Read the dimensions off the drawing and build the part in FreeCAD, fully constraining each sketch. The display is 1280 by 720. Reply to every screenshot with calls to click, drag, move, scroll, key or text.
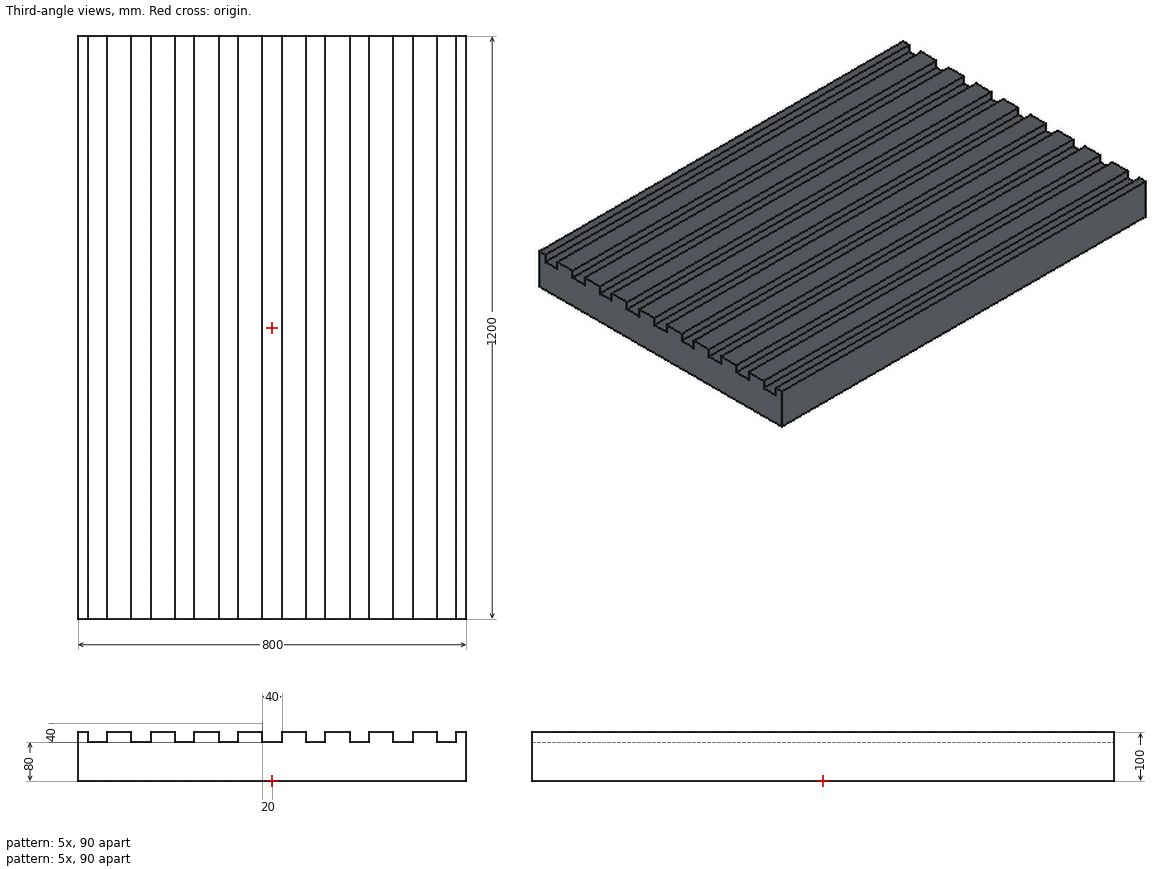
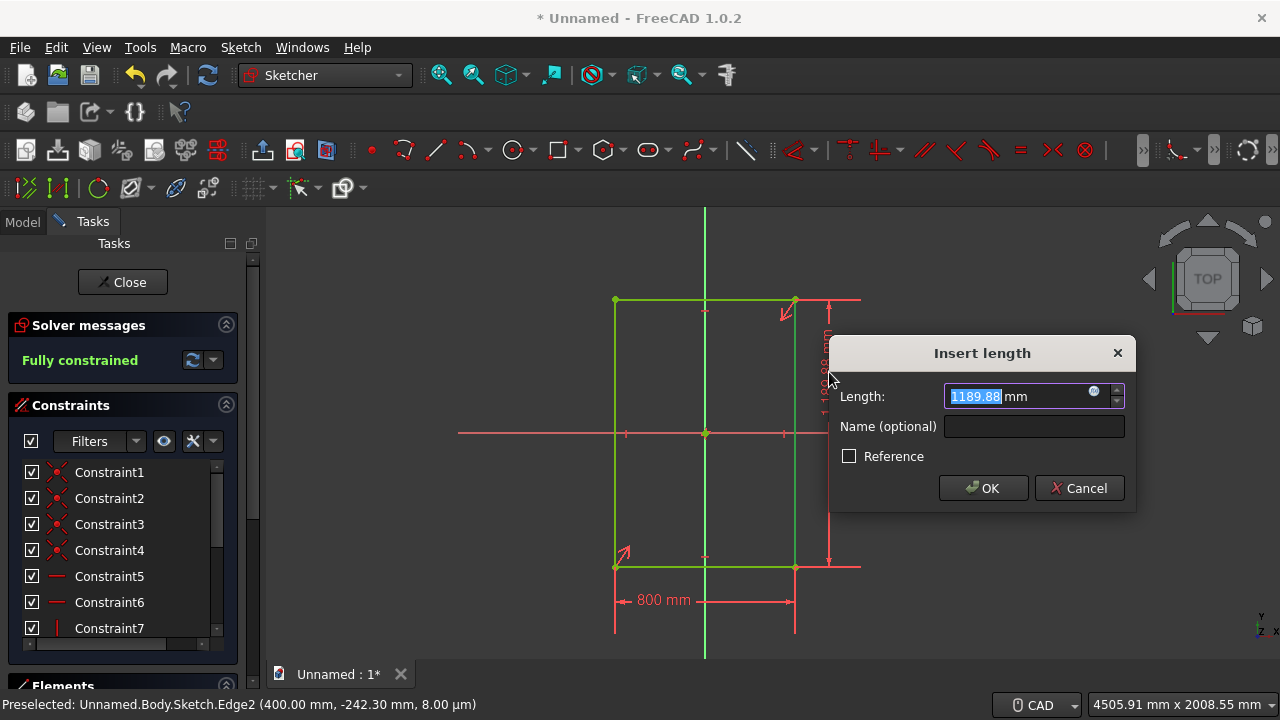
text(1200)
key(Return)
key(Escape)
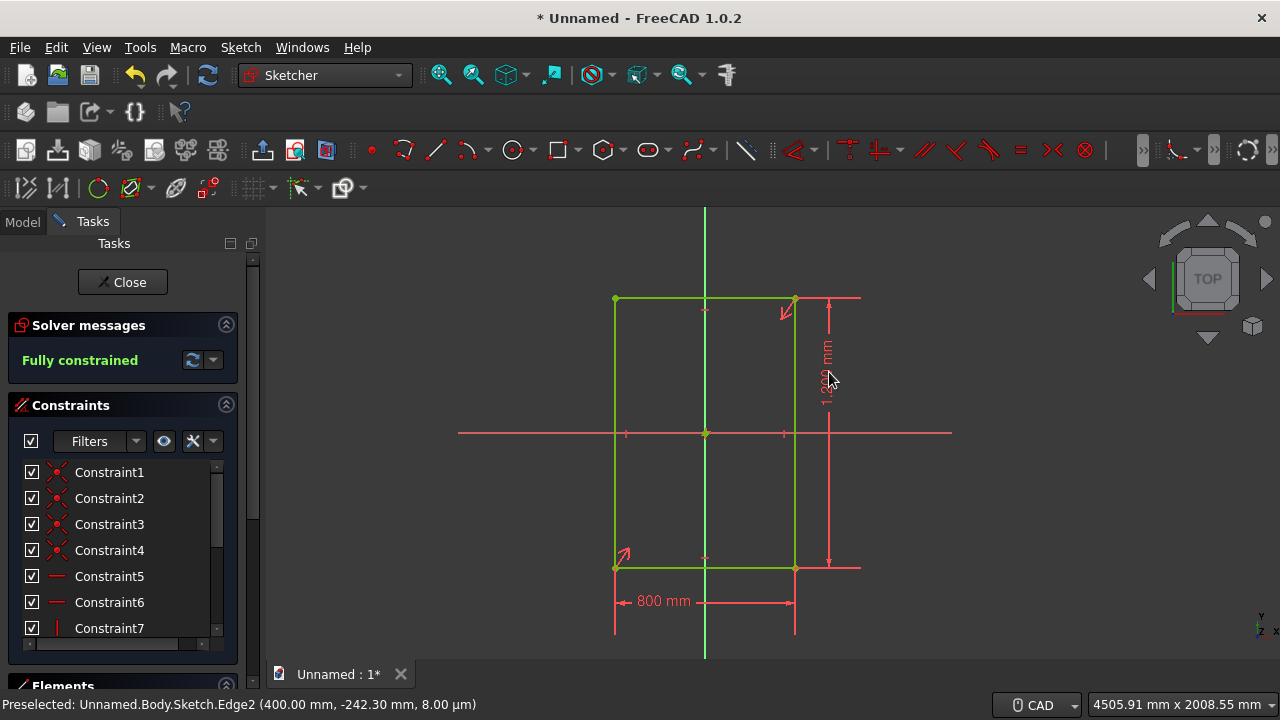
click(123, 282)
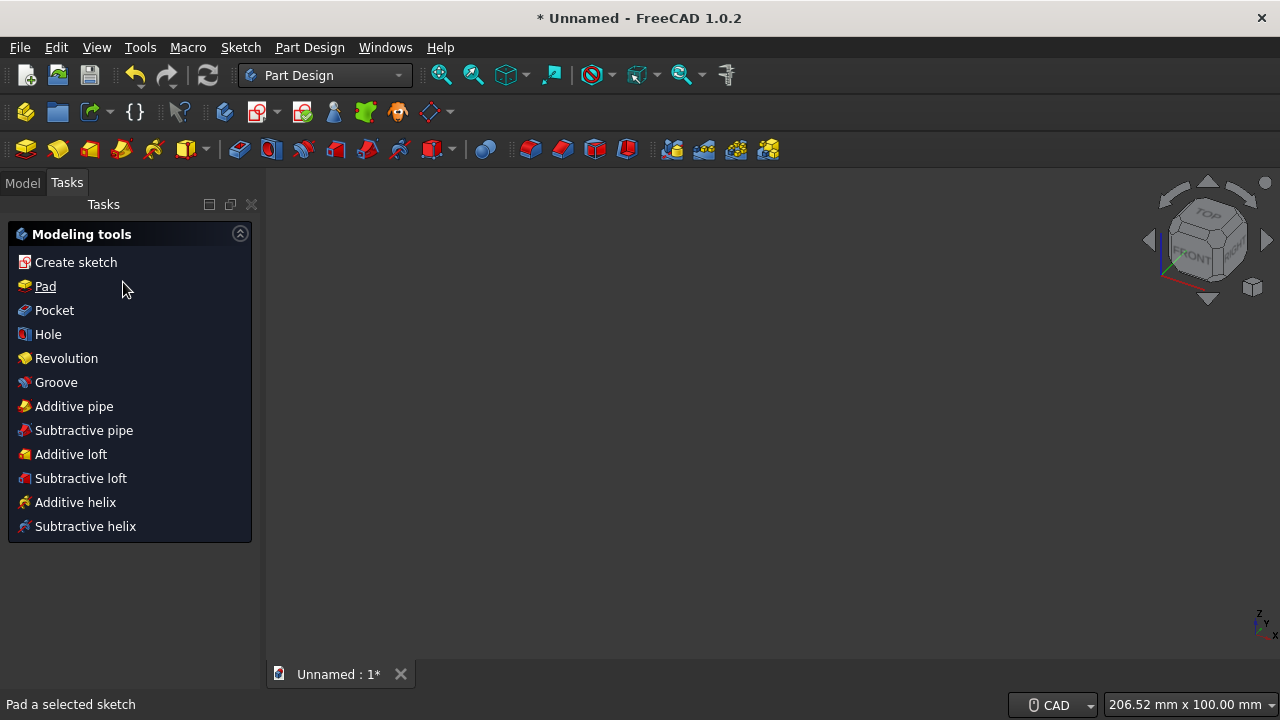
click(26, 150)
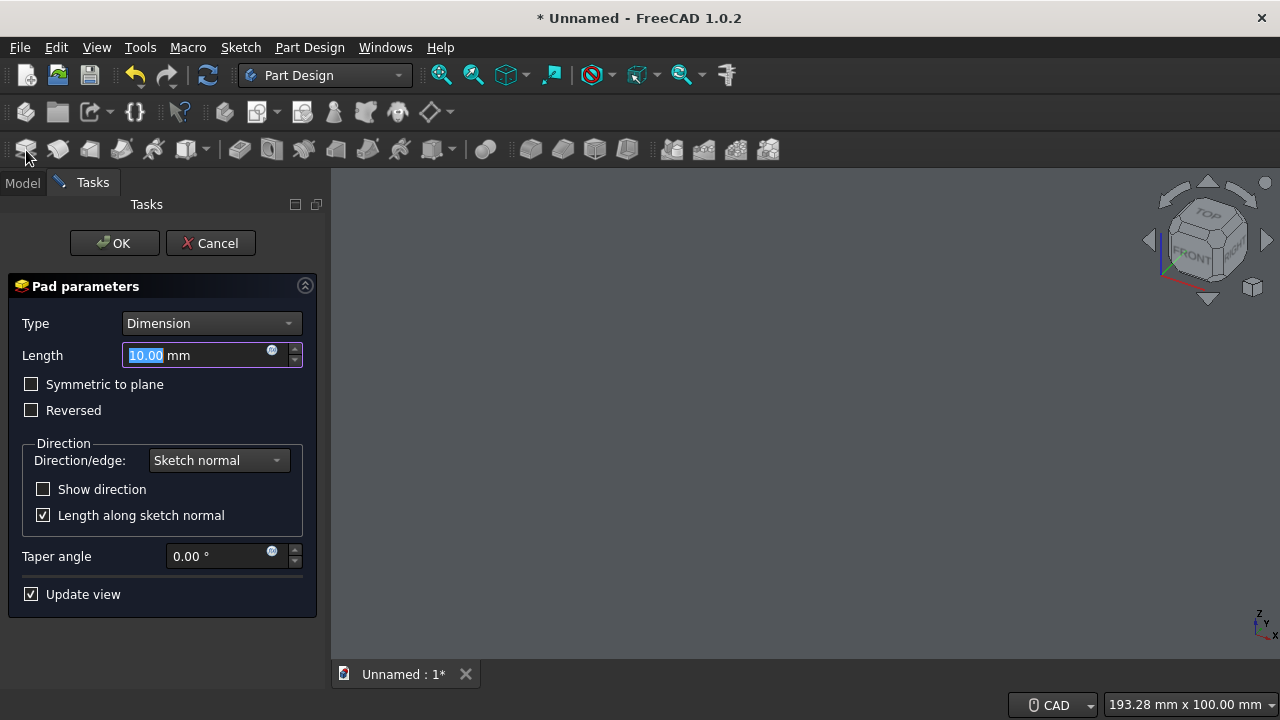
text(100)
key(Tab)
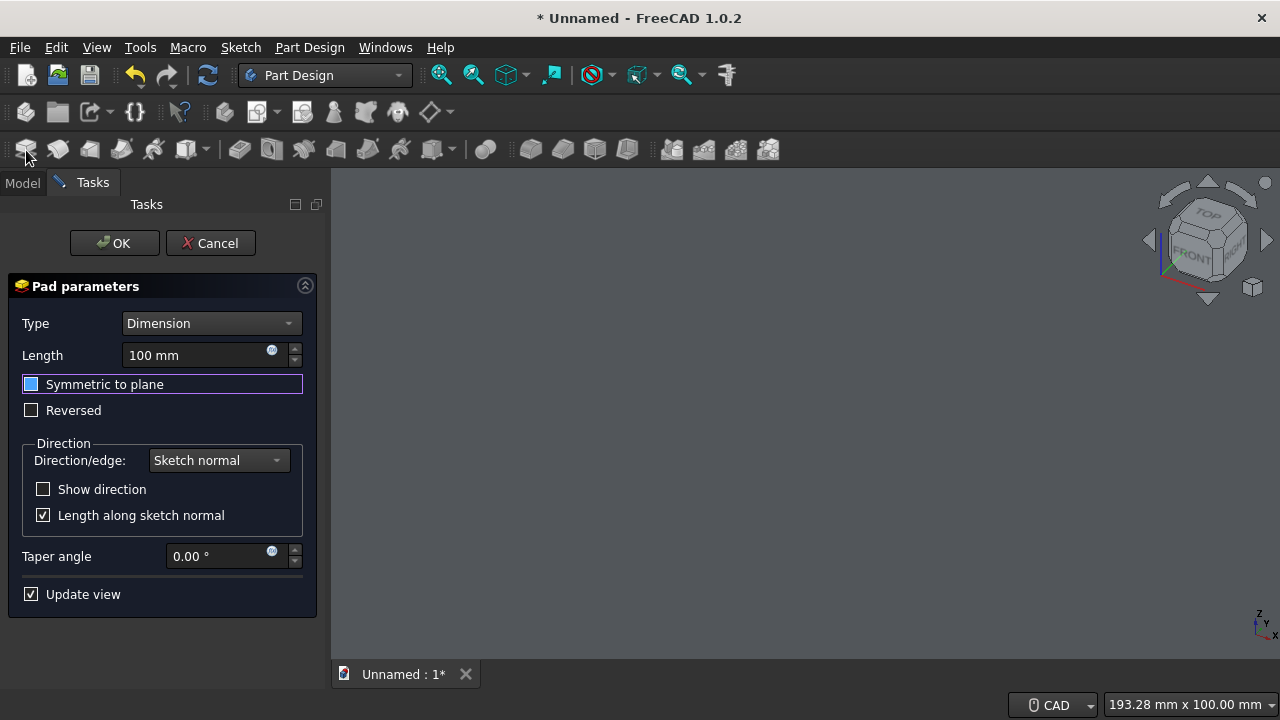
click(115, 243)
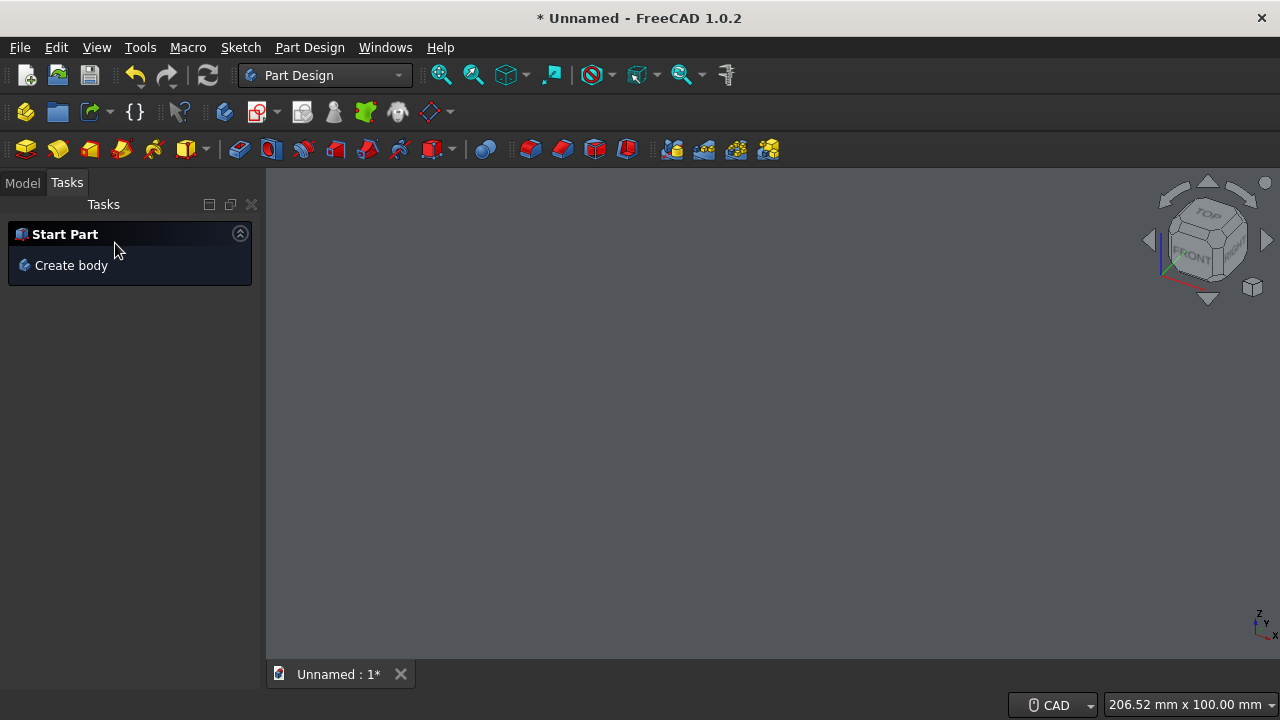
click(442, 76)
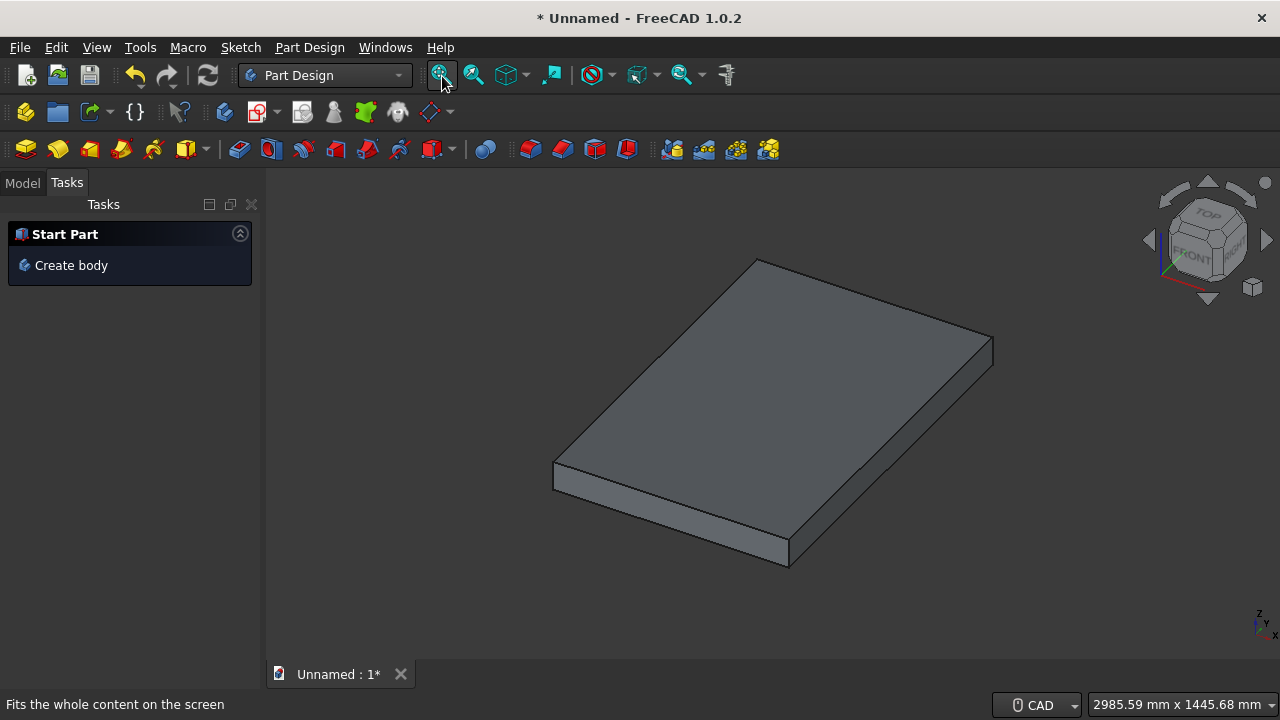
click(772, 547)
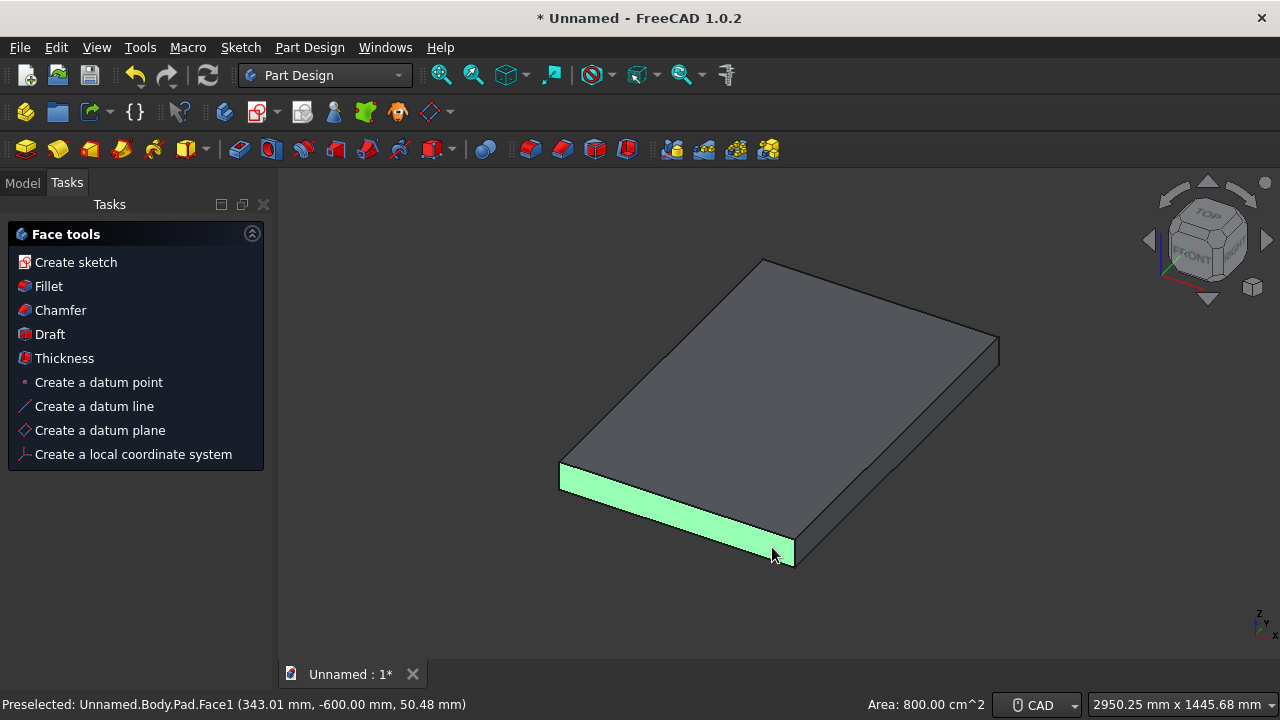
click(258, 112)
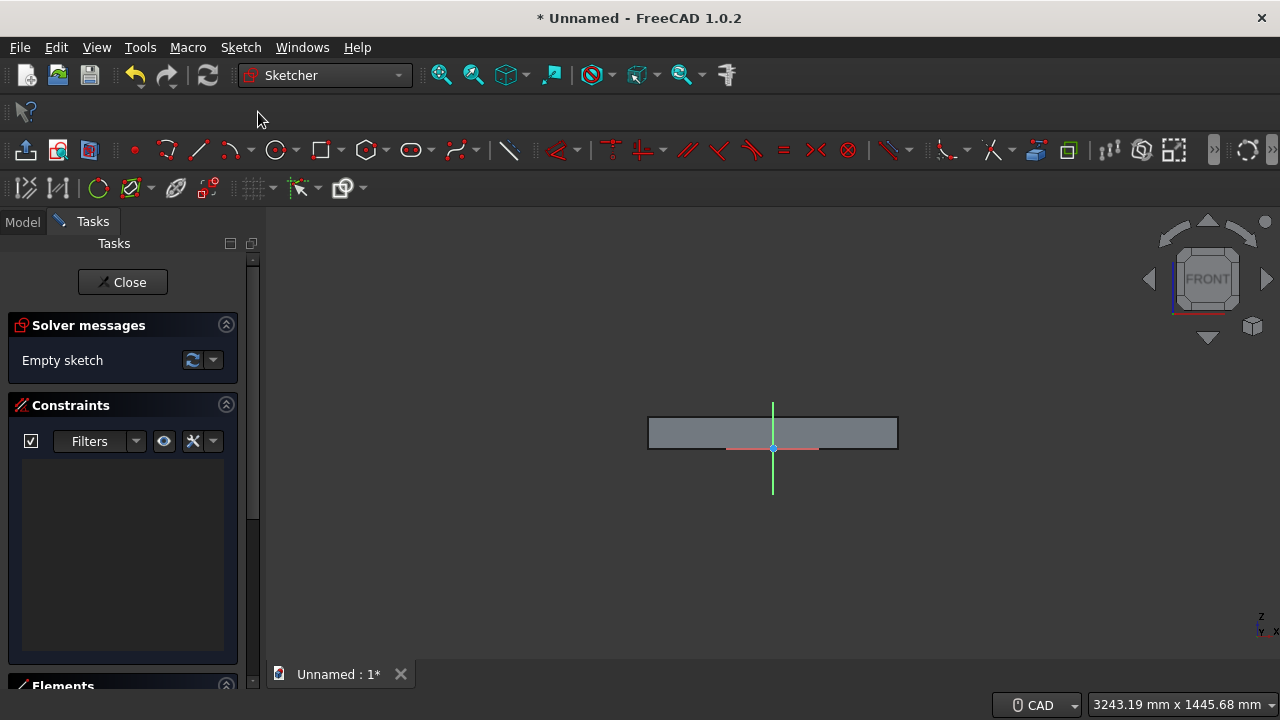
scroll(777, 417, up, 15)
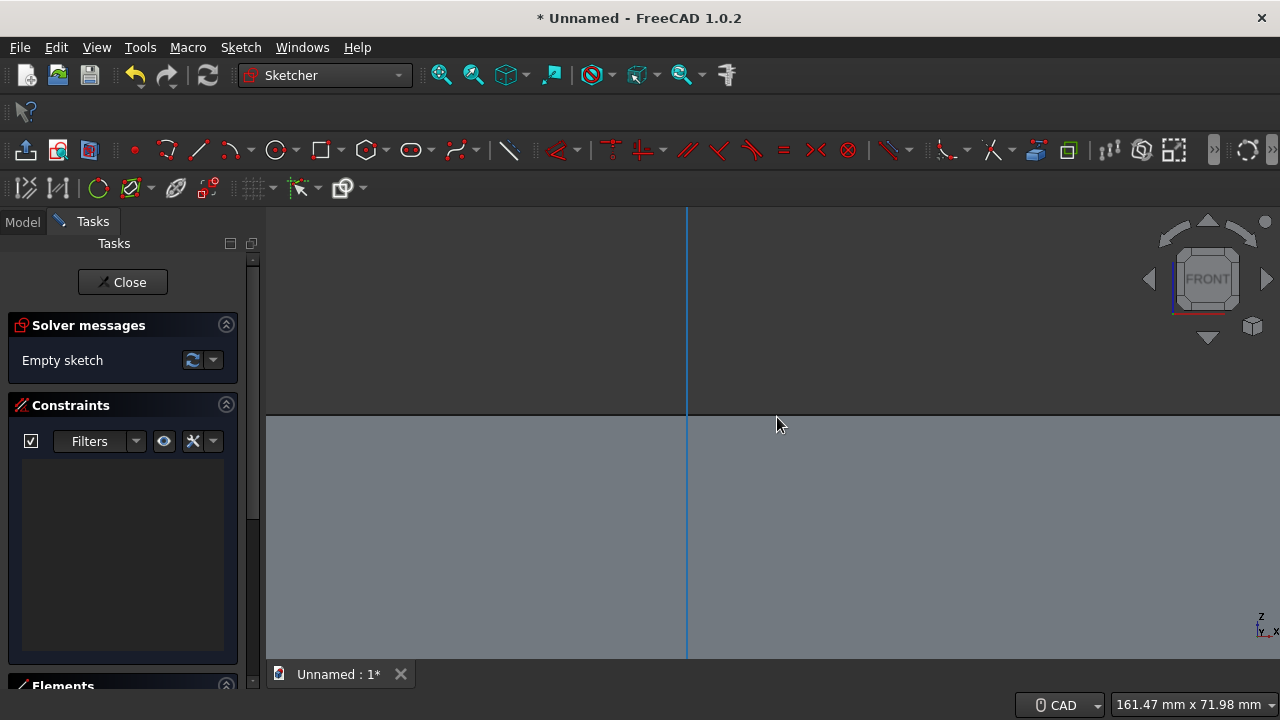
key(g)
key(r)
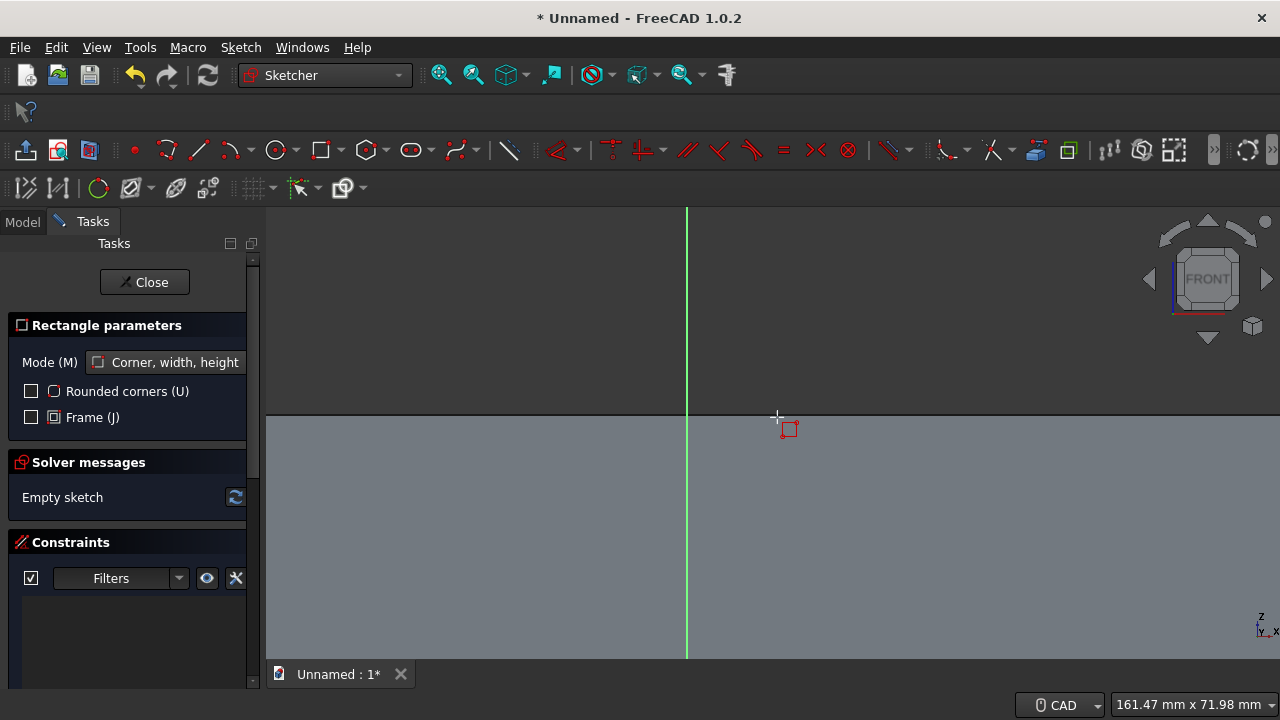
click(561, 290)
click(813, 541)
key(Escape)